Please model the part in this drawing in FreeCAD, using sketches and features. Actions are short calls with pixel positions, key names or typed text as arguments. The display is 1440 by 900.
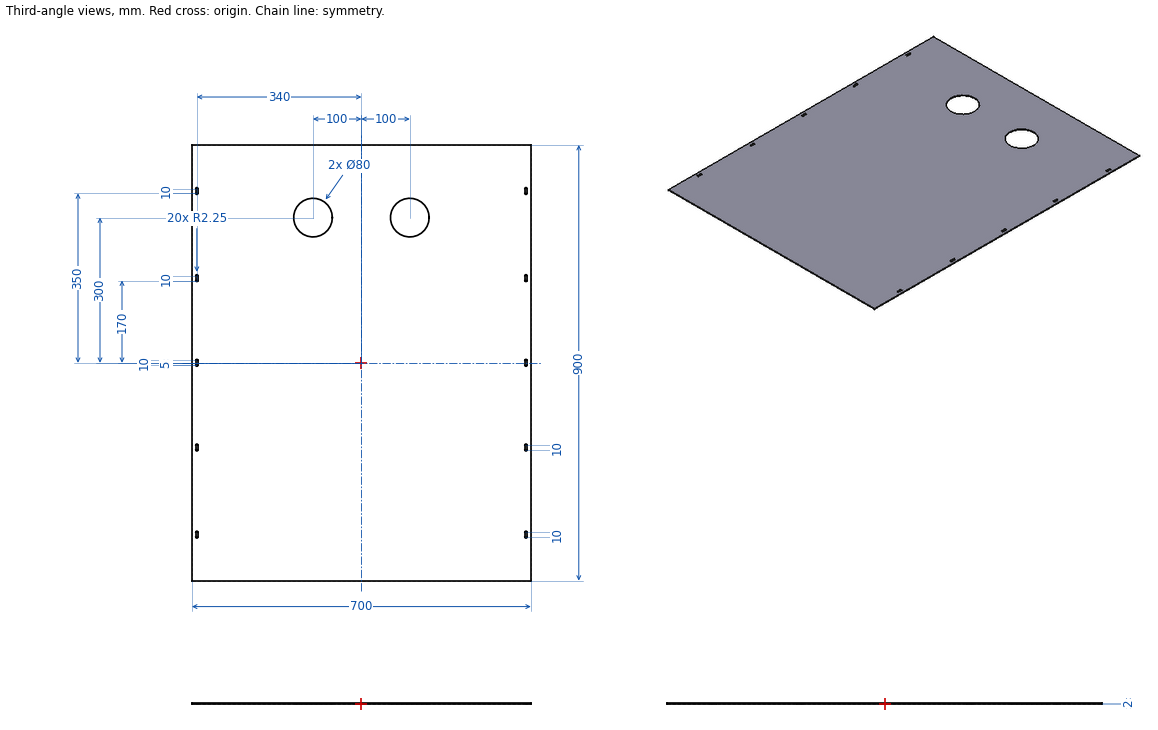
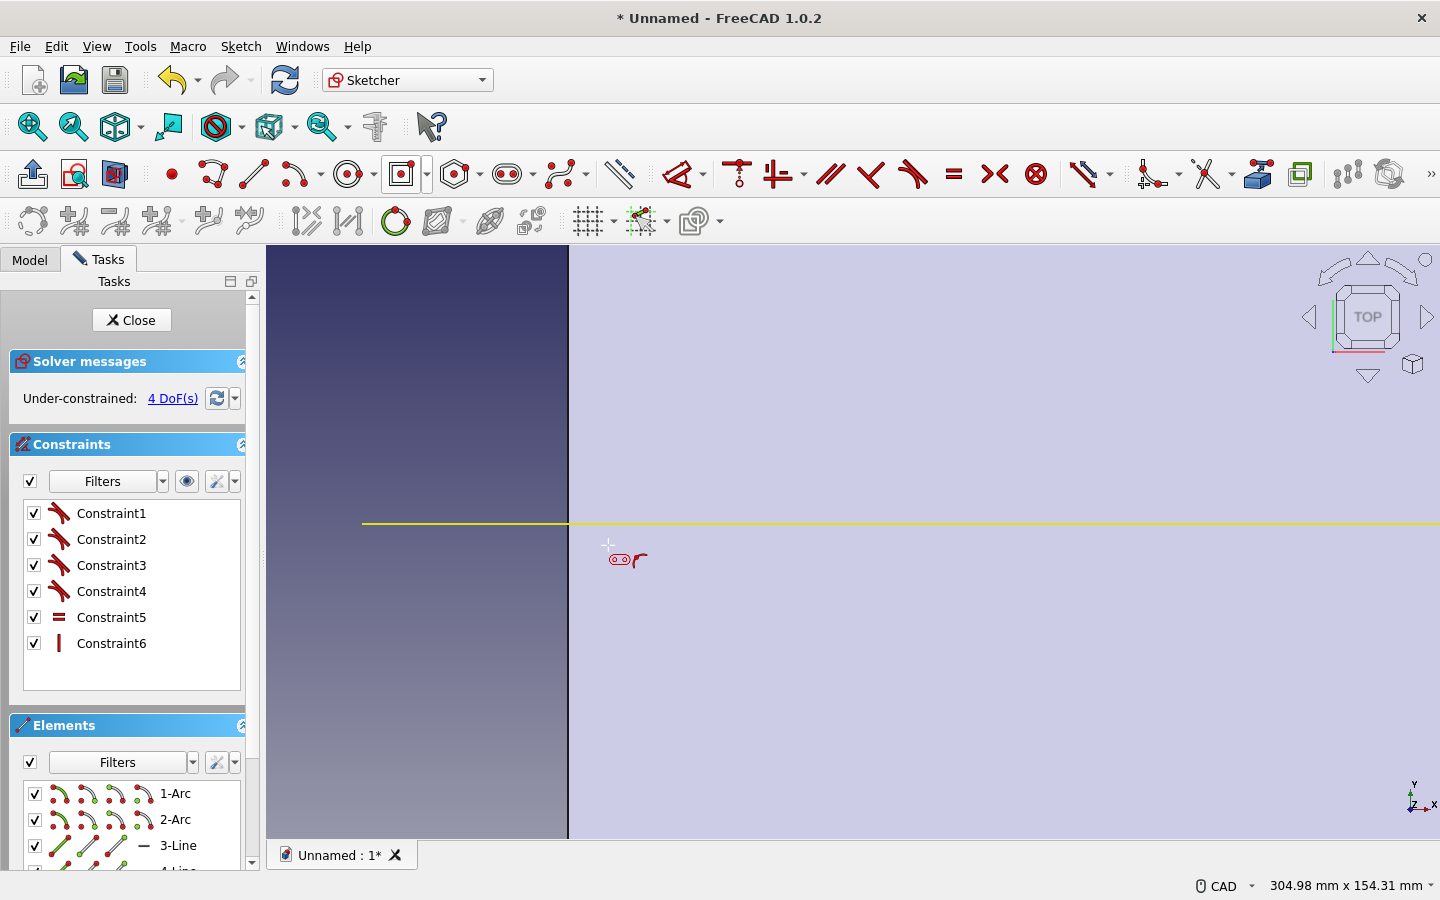
click(607, 544)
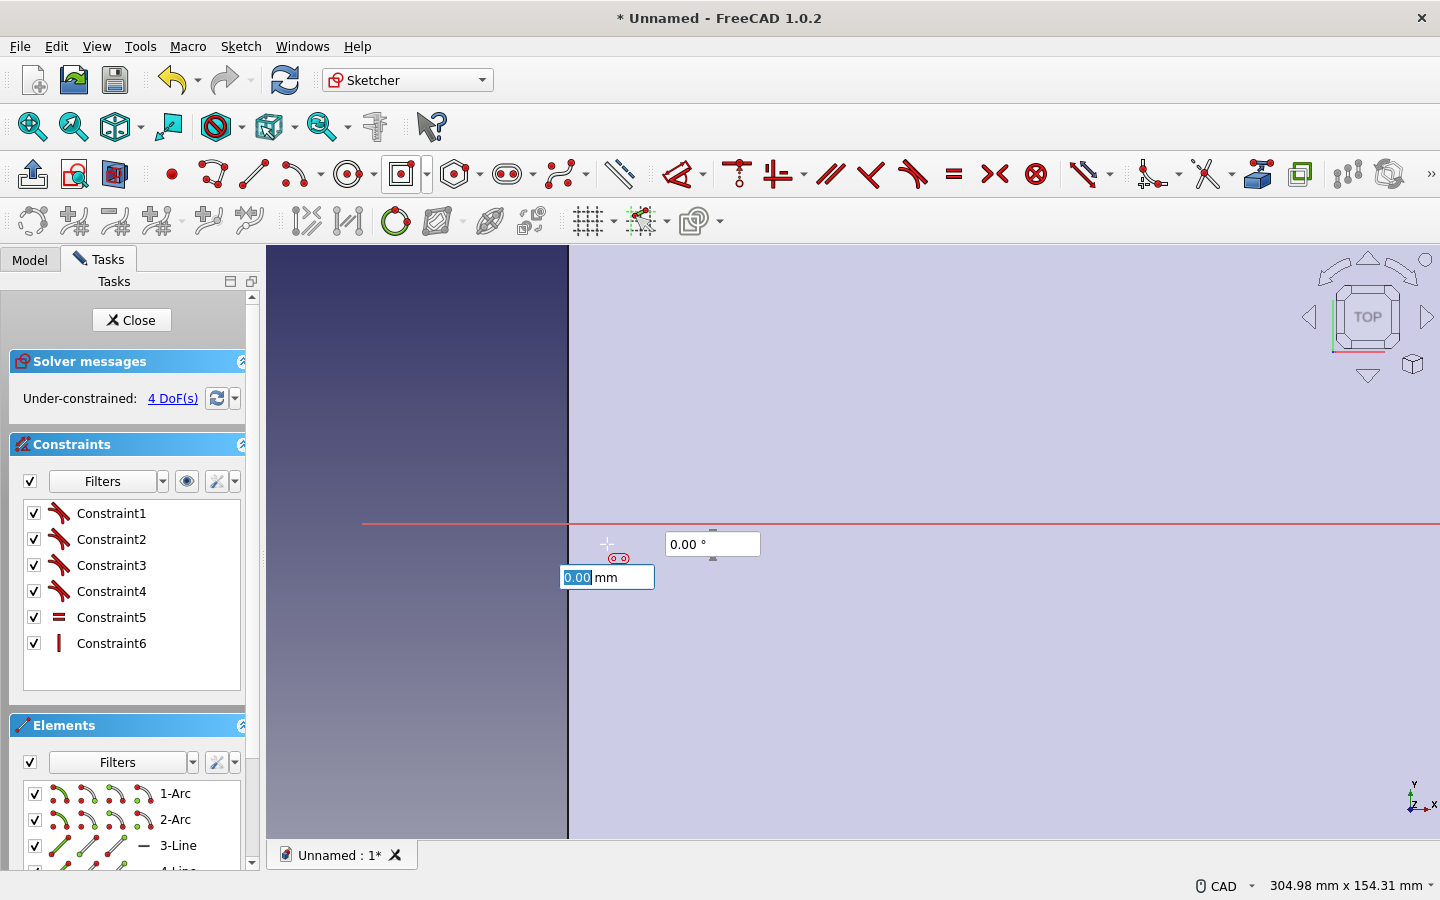
click(607, 505)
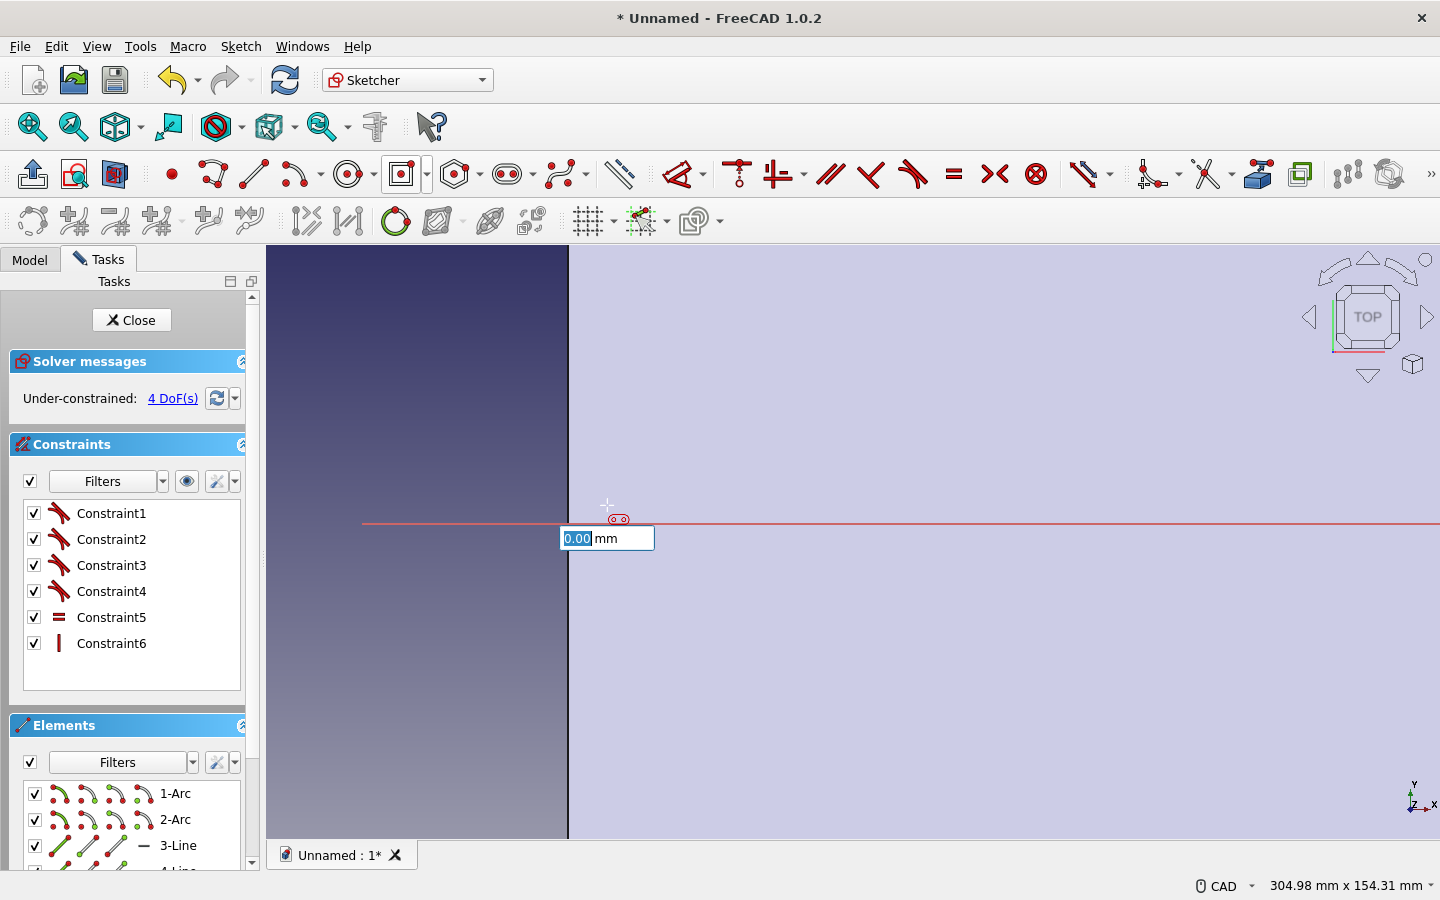
scroll(598, 519, up, 6)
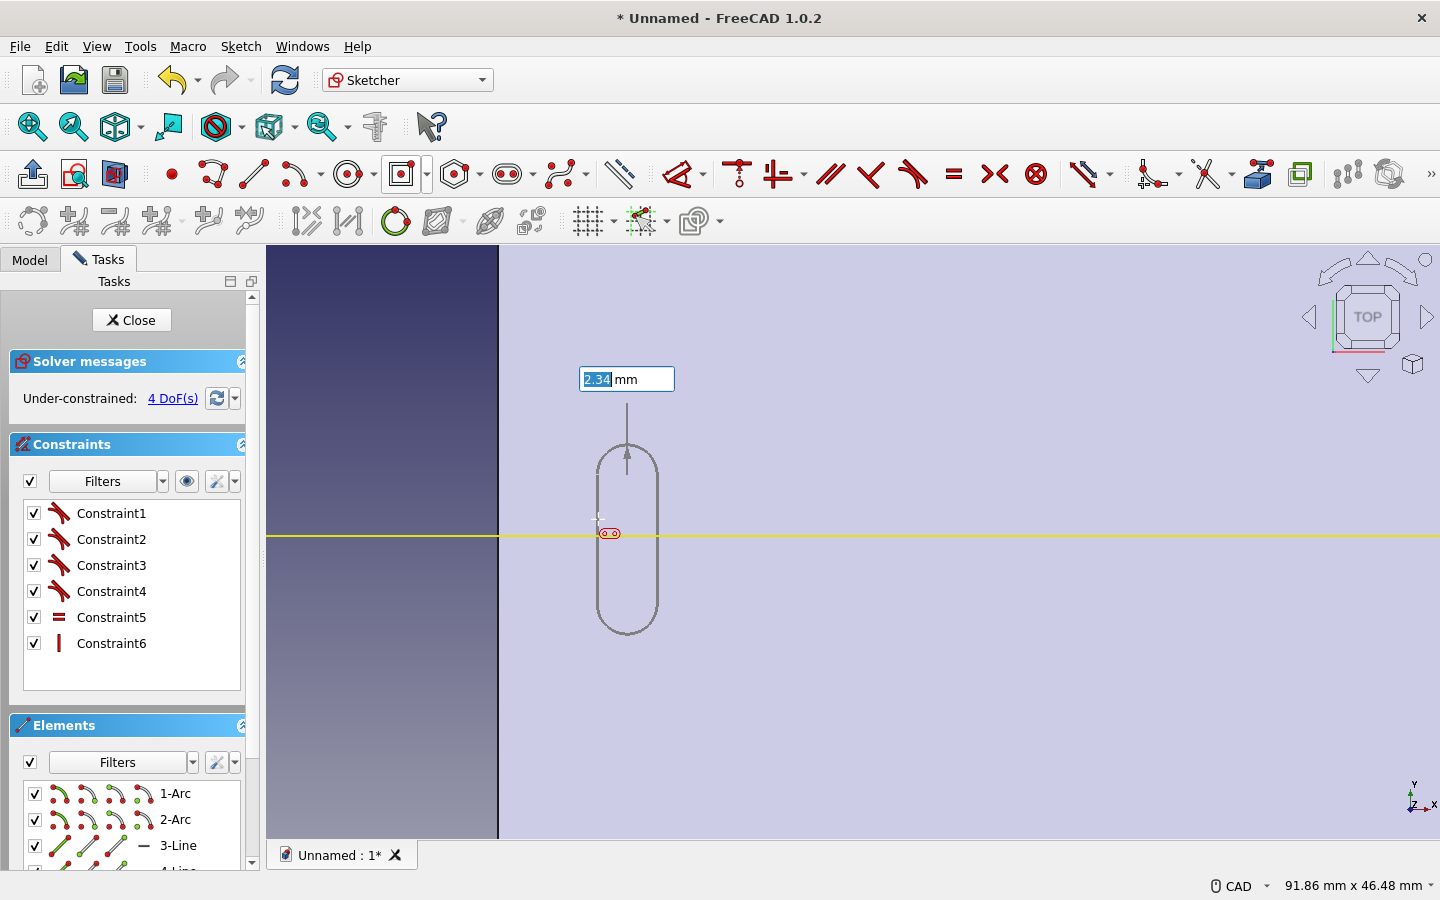
click(597, 517)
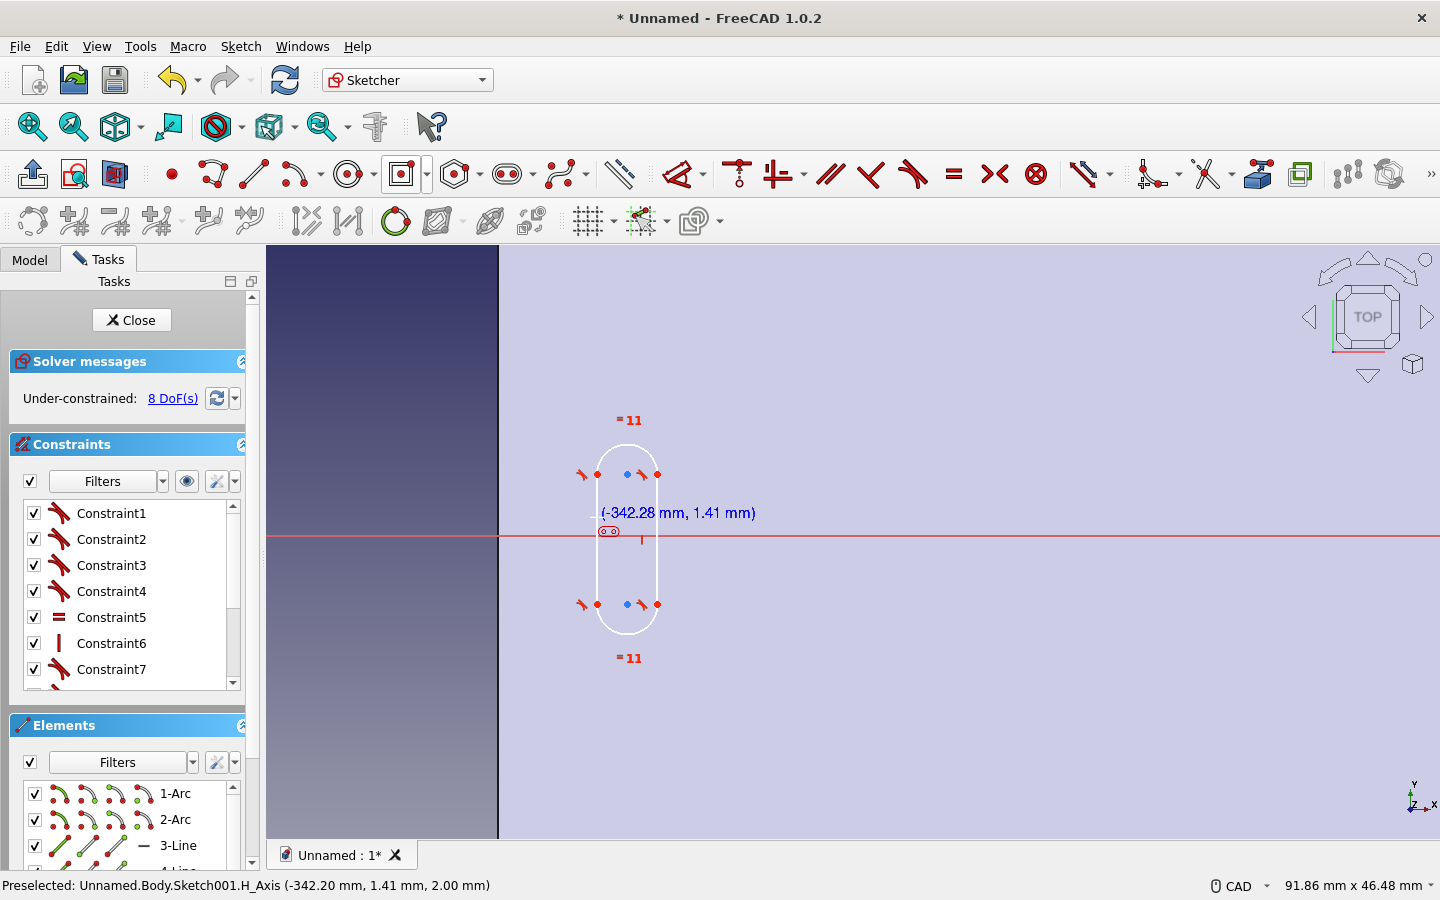
scroll(565, 542, down, 15)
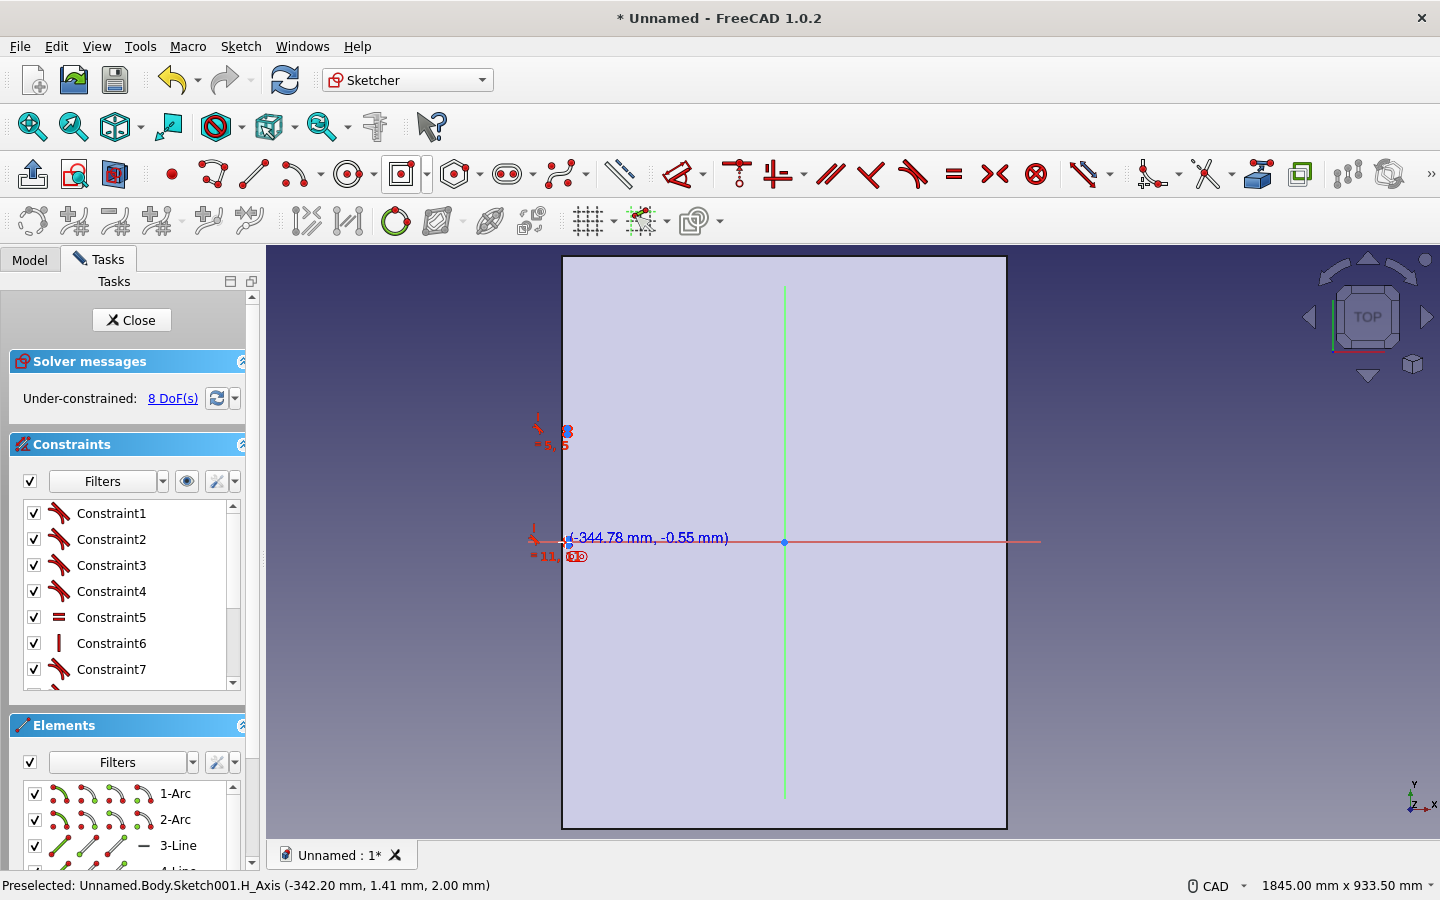
scroll(1001, 434, up, 14)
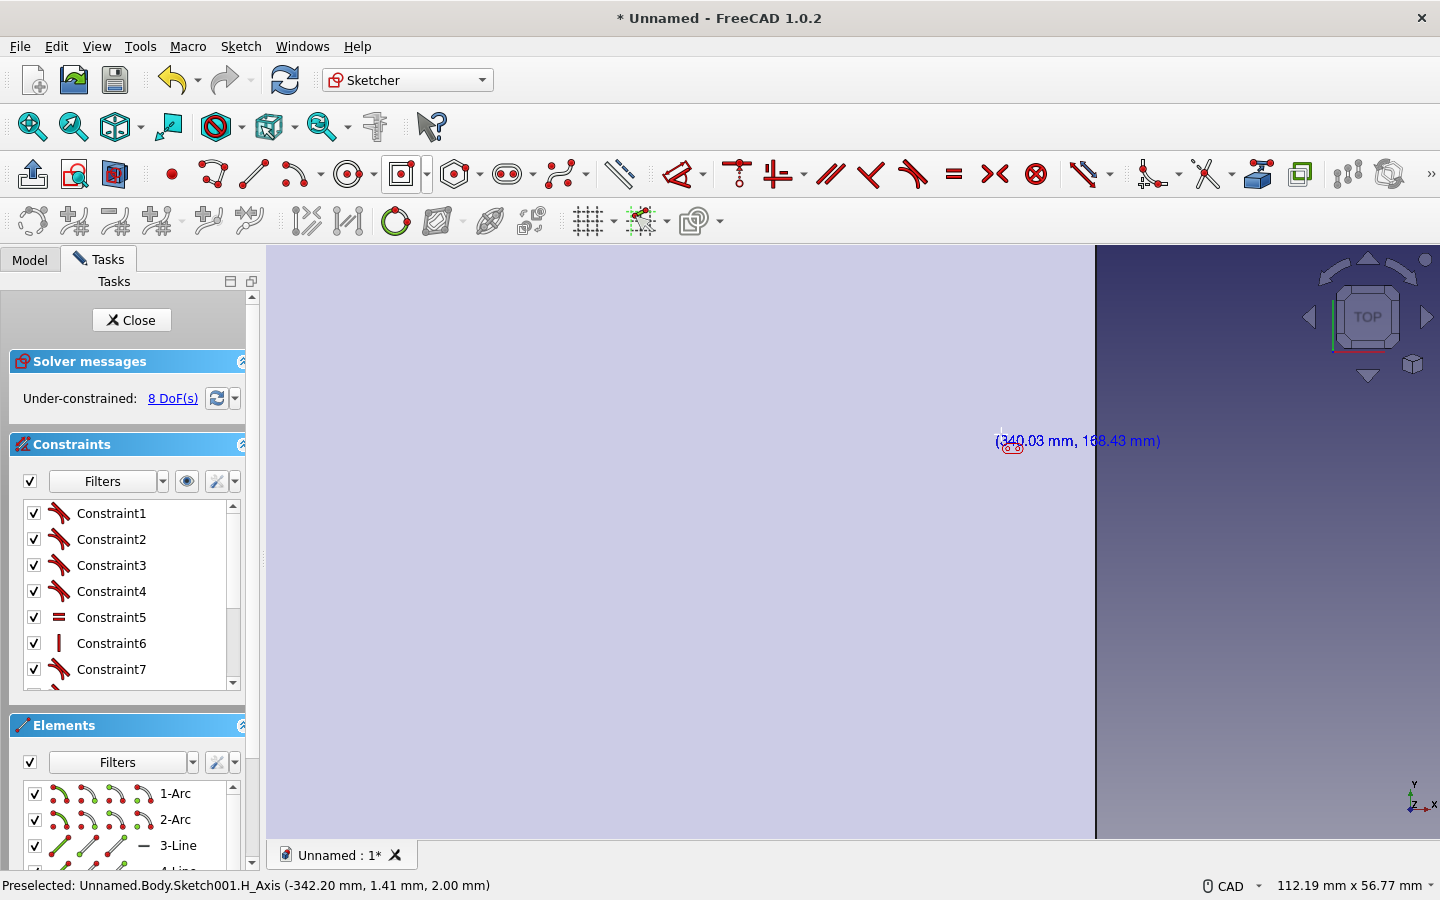
scroll(960, 455, down, 15)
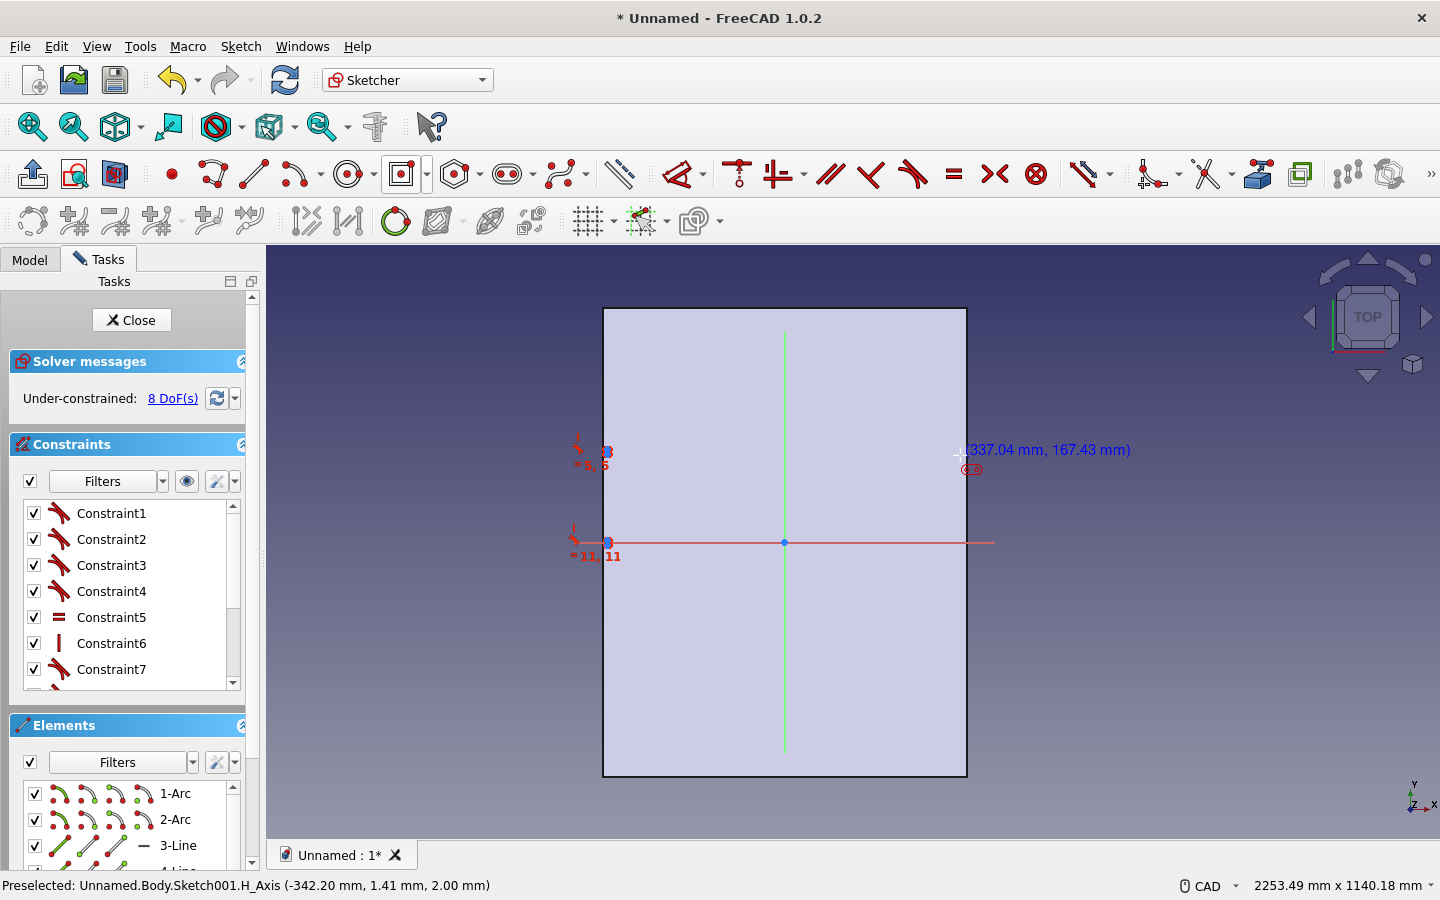
click(962, 454)